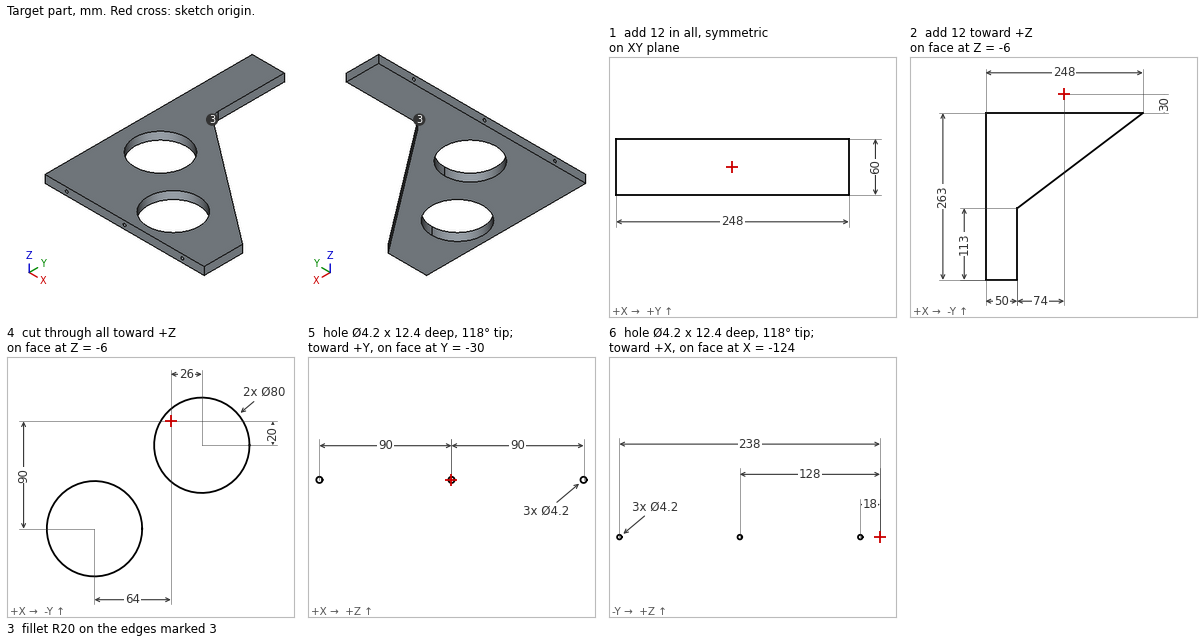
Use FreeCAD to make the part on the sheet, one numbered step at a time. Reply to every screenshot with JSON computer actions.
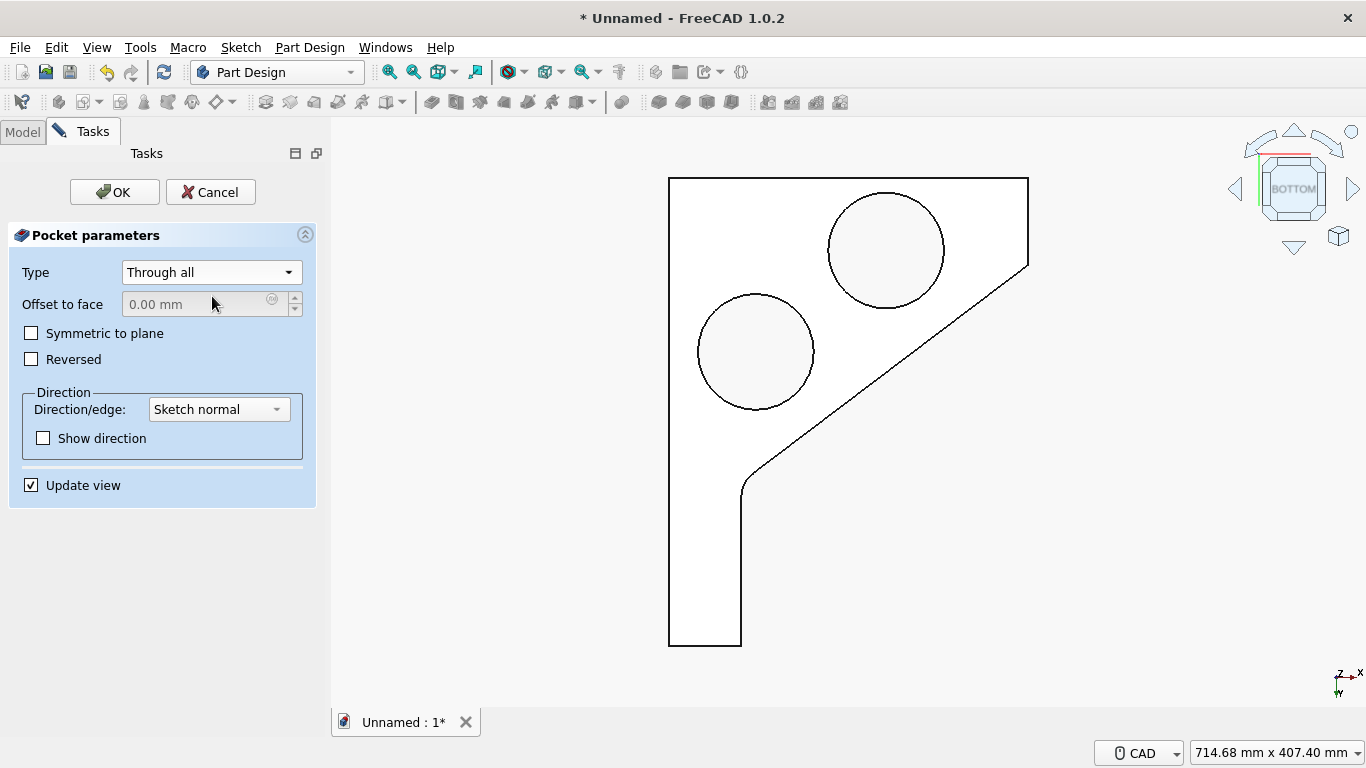
{"action": "left_click", "coordinate": [115, 192]}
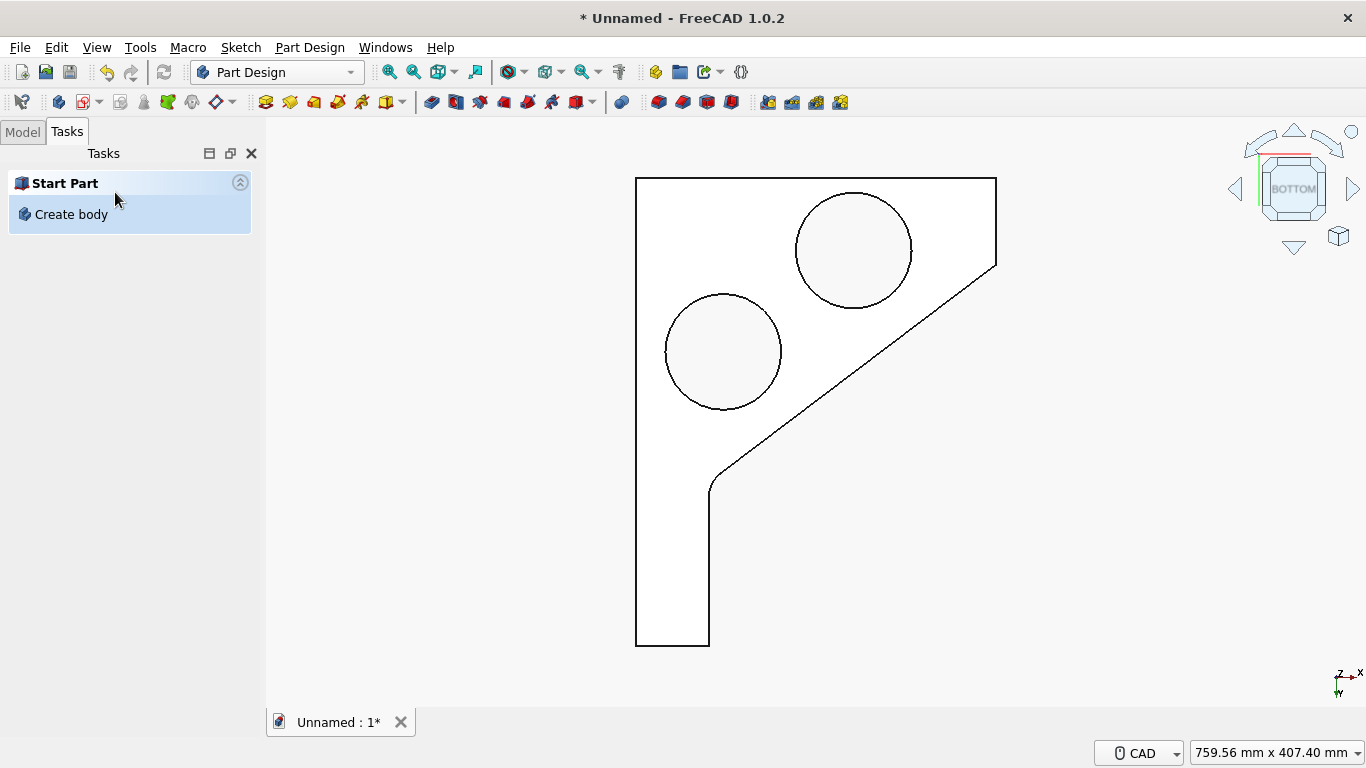
{"action": "key", "text": "0"}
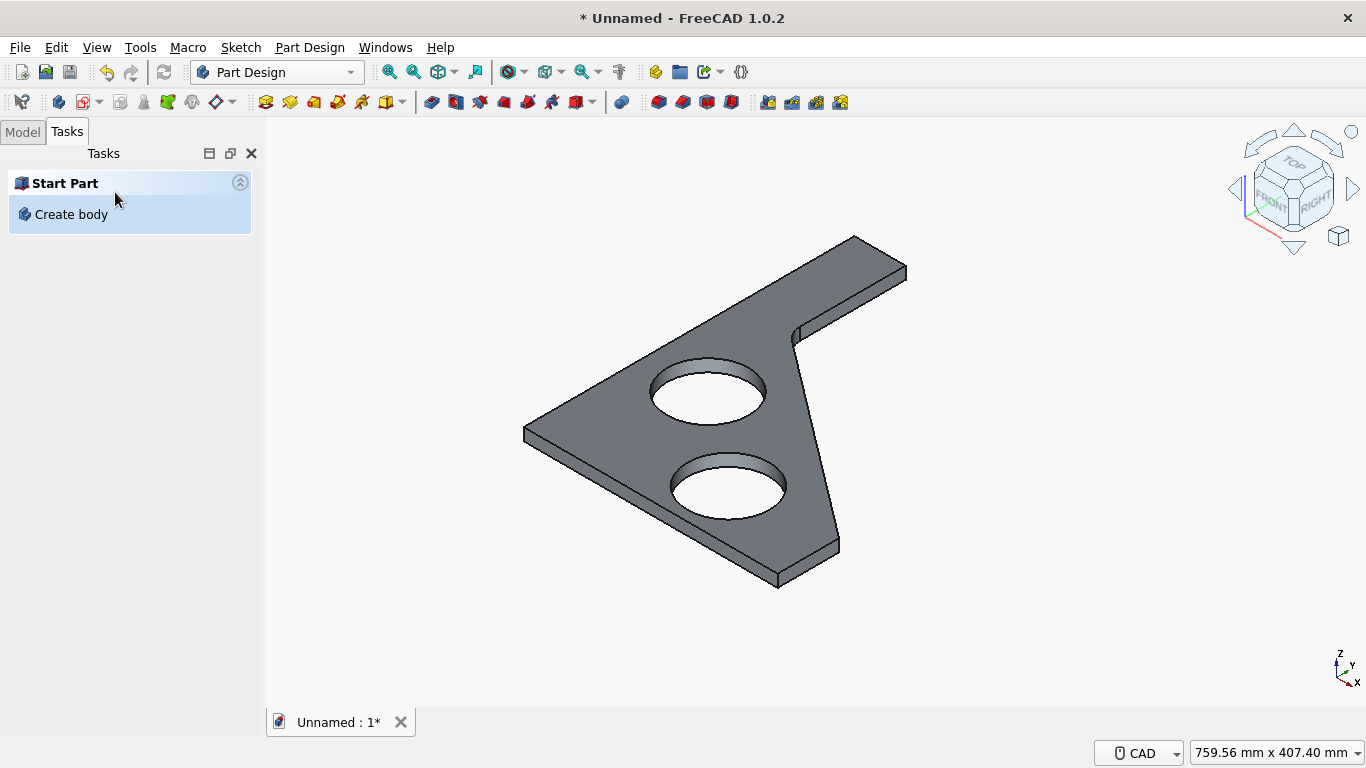
{"action": "key", "text": "1"}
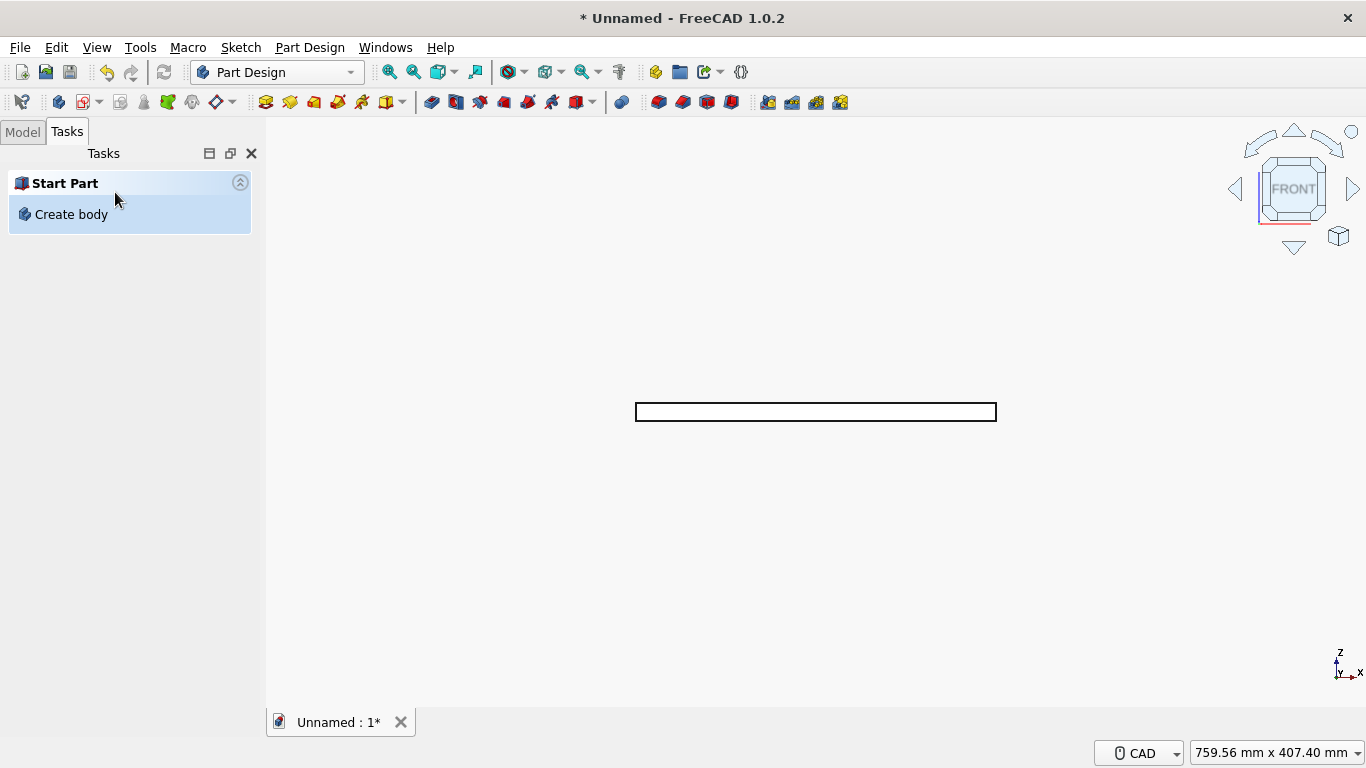
{"action": "key", "text": "v f"}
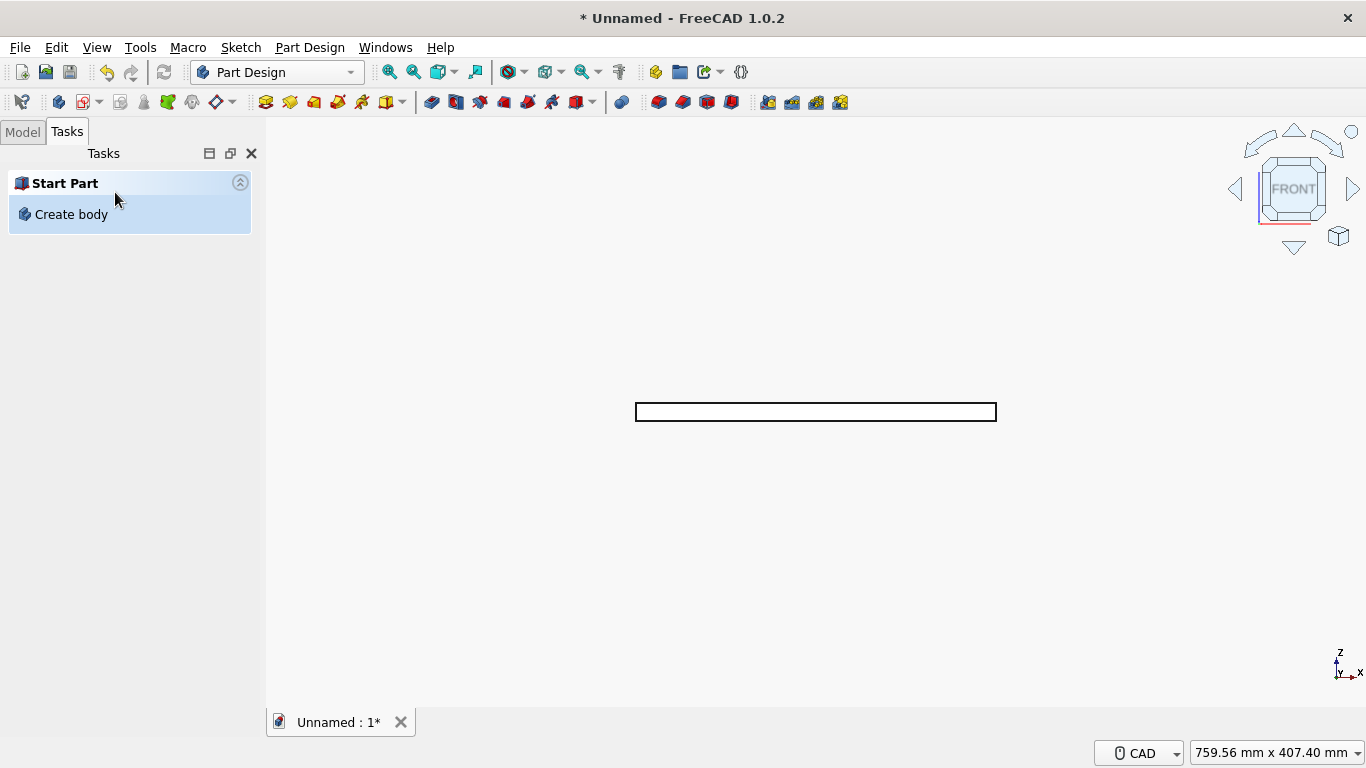
{"action": "left_click", "coordinate": [970, 411]}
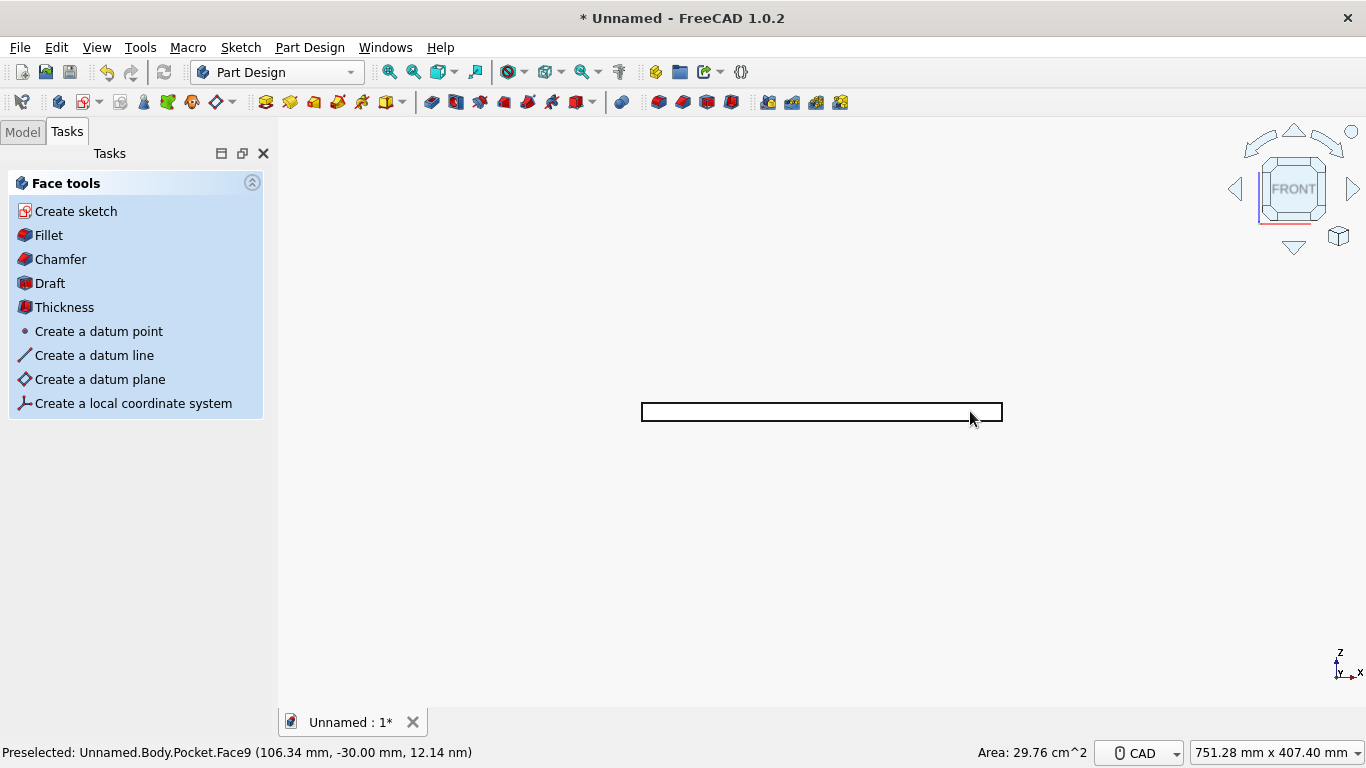
{"action": "left_click", "coordinate": [84, 102]}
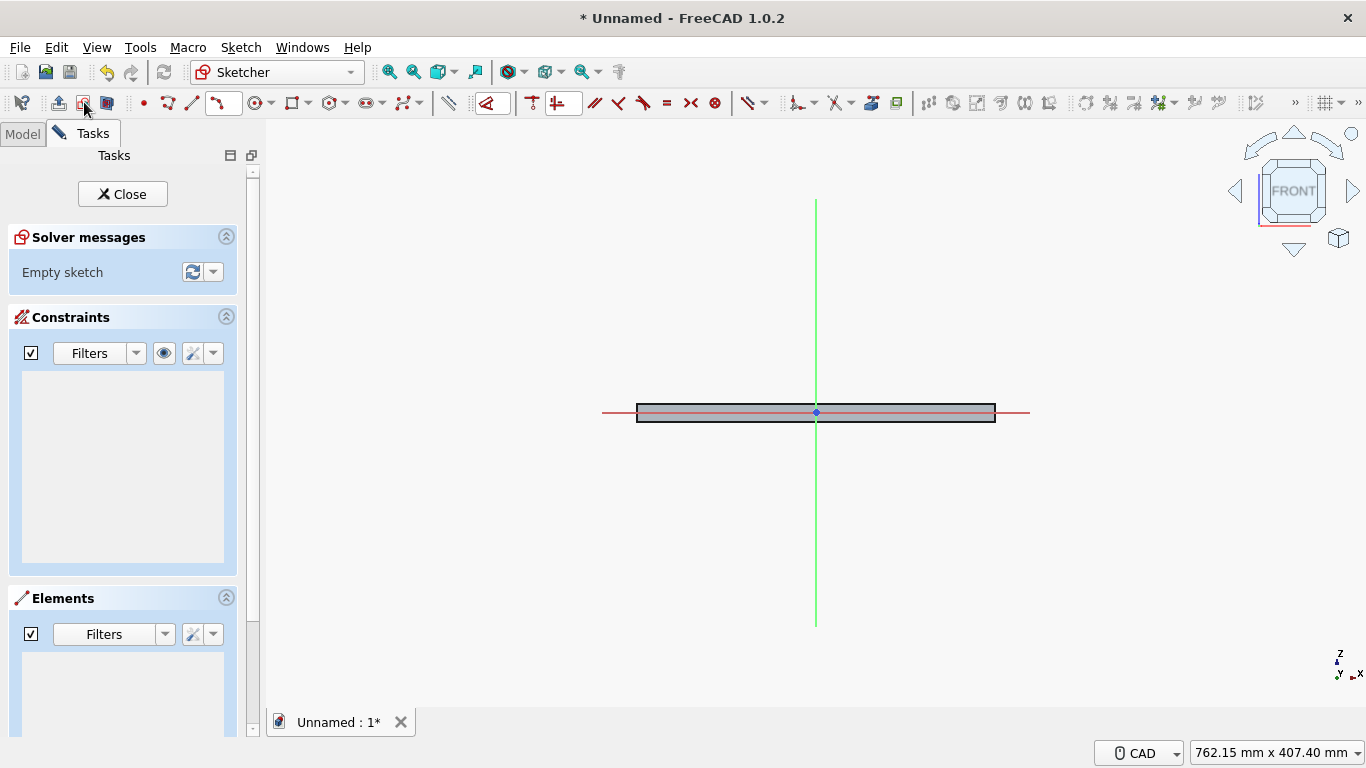
{"action": "scroll", "coordinate": [872, 413], "scroll_direction": "up", "scroll_amount": 4}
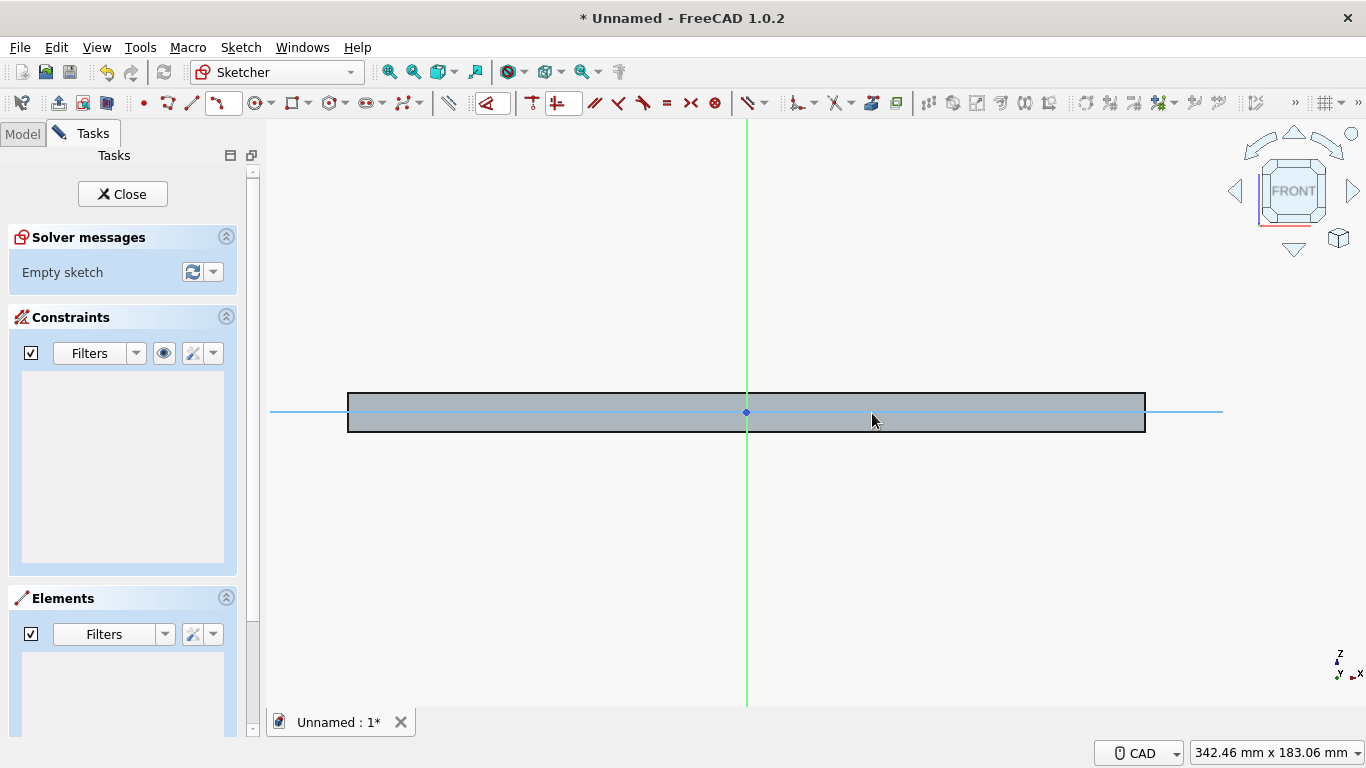
{"action": "key", "text": "g c"}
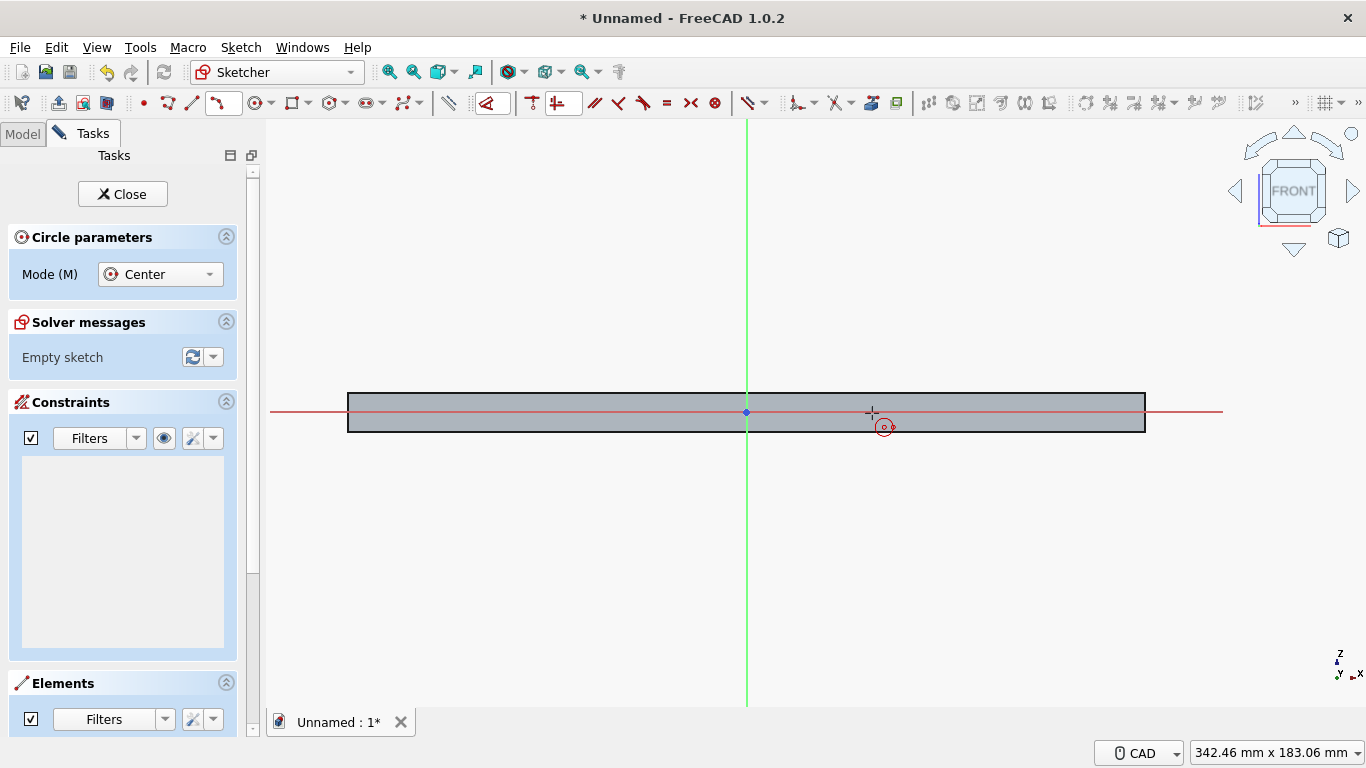
{"action": "scroll", "coordinate": [1036, 412], "scroll_direction": "up", "scroll_amount": 7}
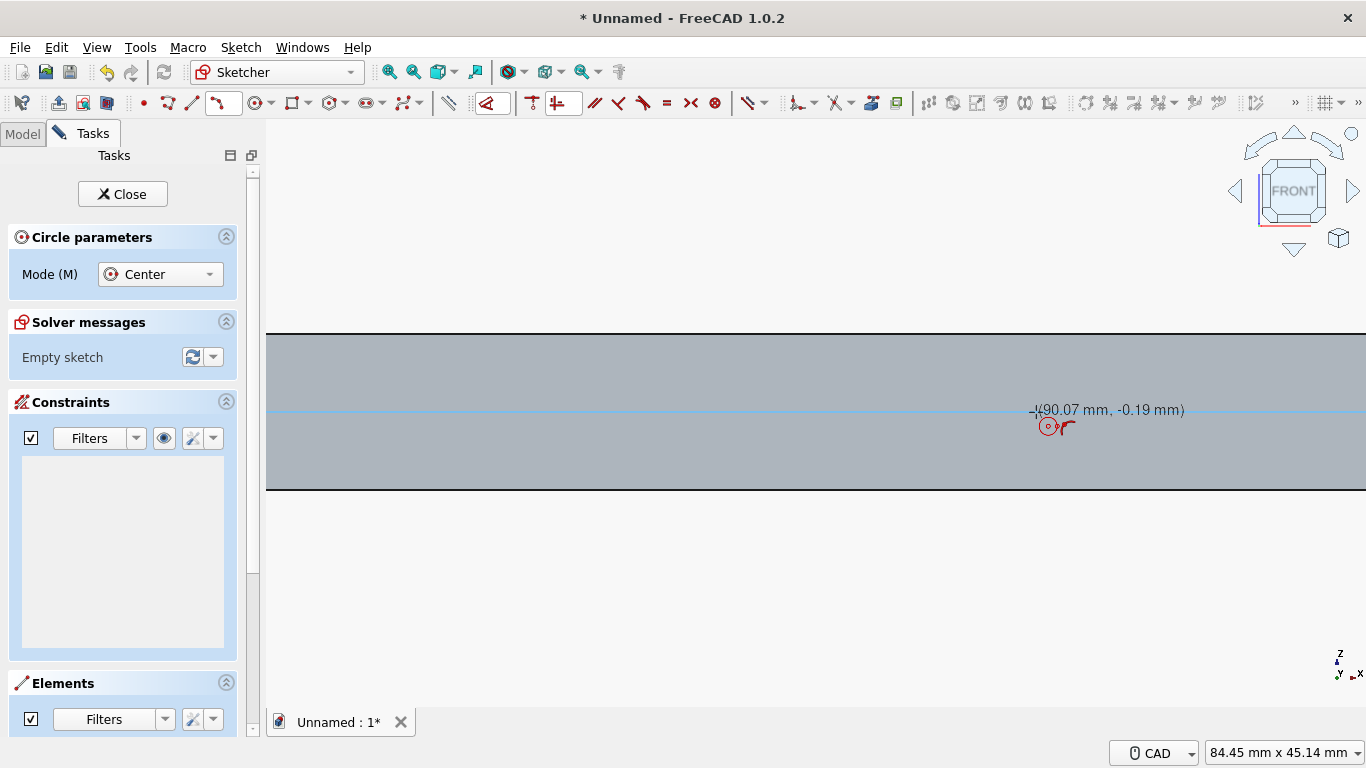
{"action": "scroll", "coordinate": [1038, 413], "scroll_direction": "down", "scroll_amount": 7}